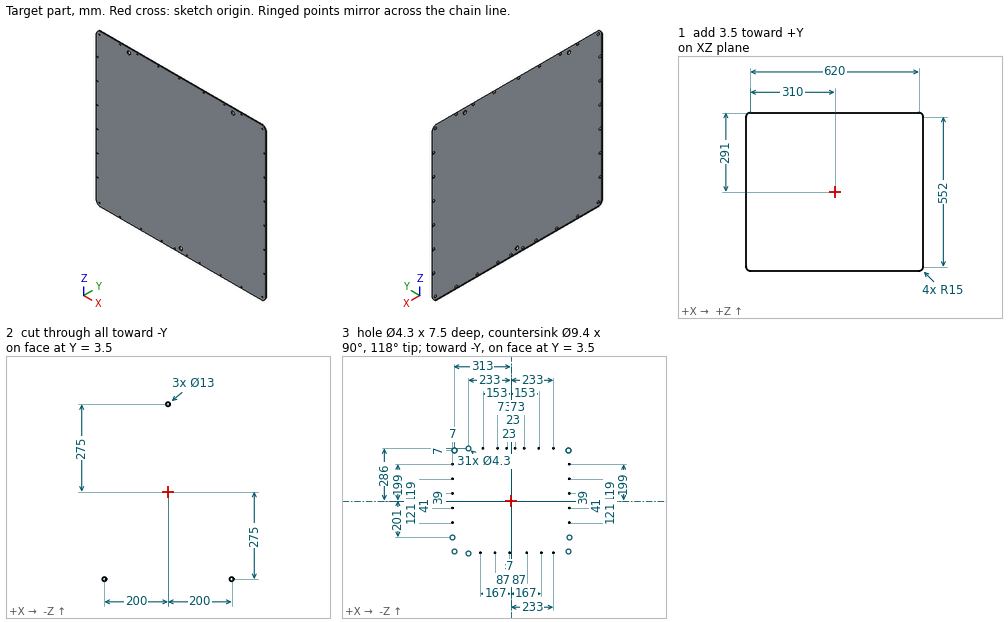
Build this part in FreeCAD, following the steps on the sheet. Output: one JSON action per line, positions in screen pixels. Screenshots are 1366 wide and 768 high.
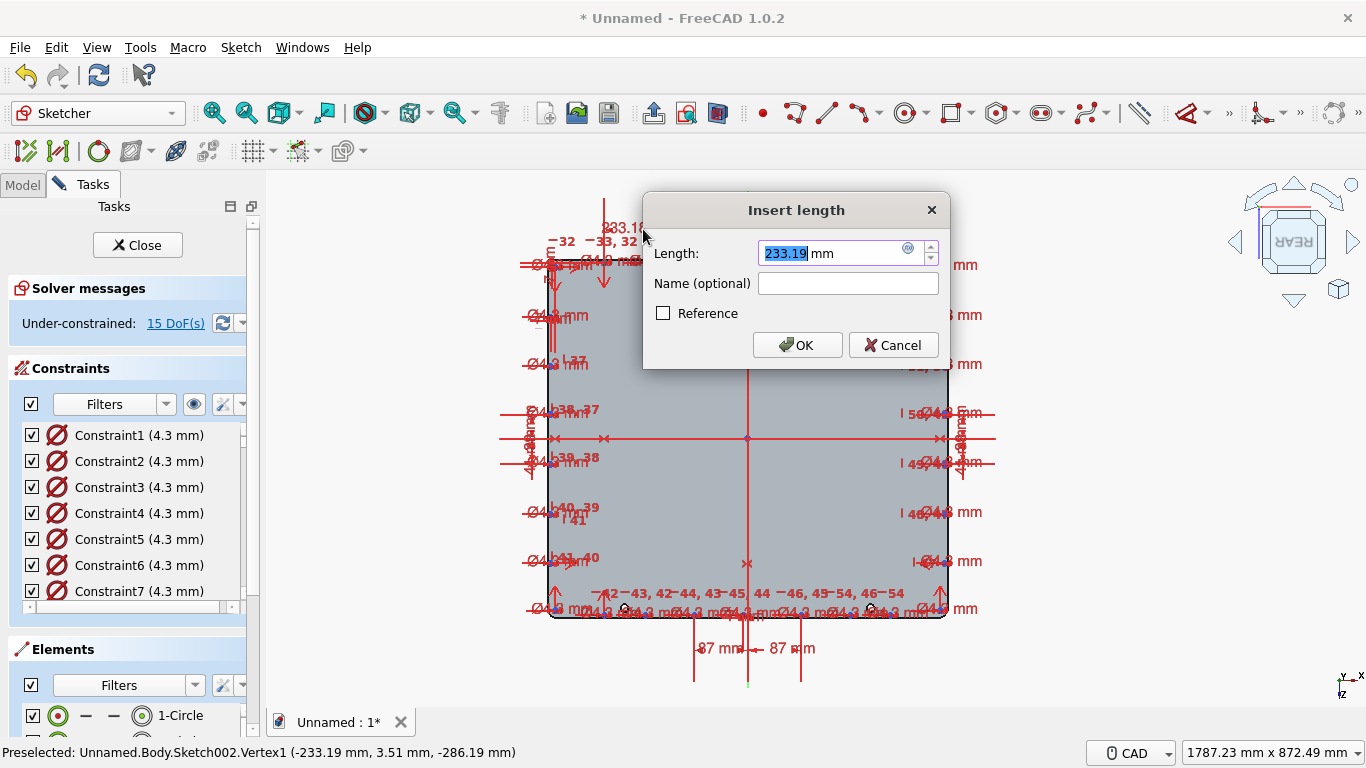
{"action": "type", "text": "233"}
{"action": "key", "text": "Return"}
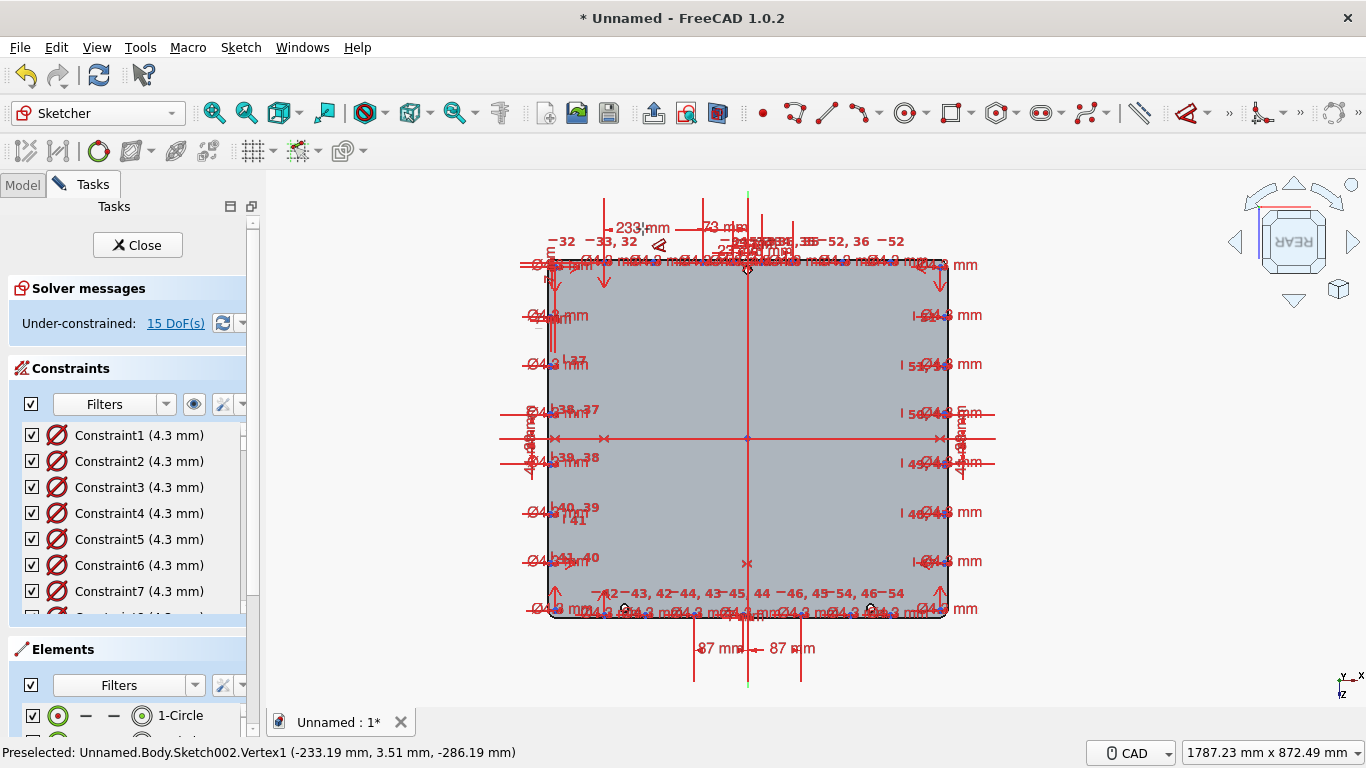
{"action": "left_click", "coordinate": [604, 263]}
{"action": "left_click", "coordinate": [570, 351]}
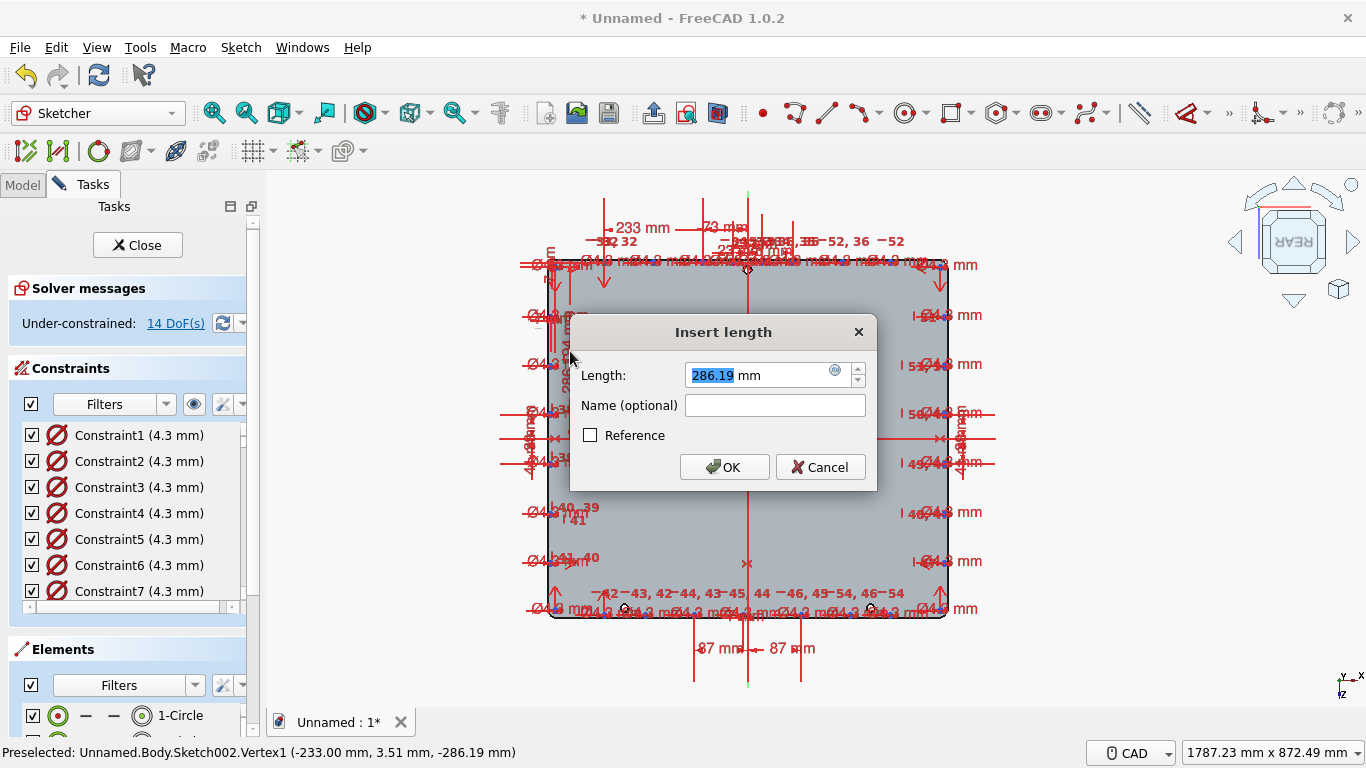
{"action": "type", "text": "286"}
{"action": "key", "text": "Return"}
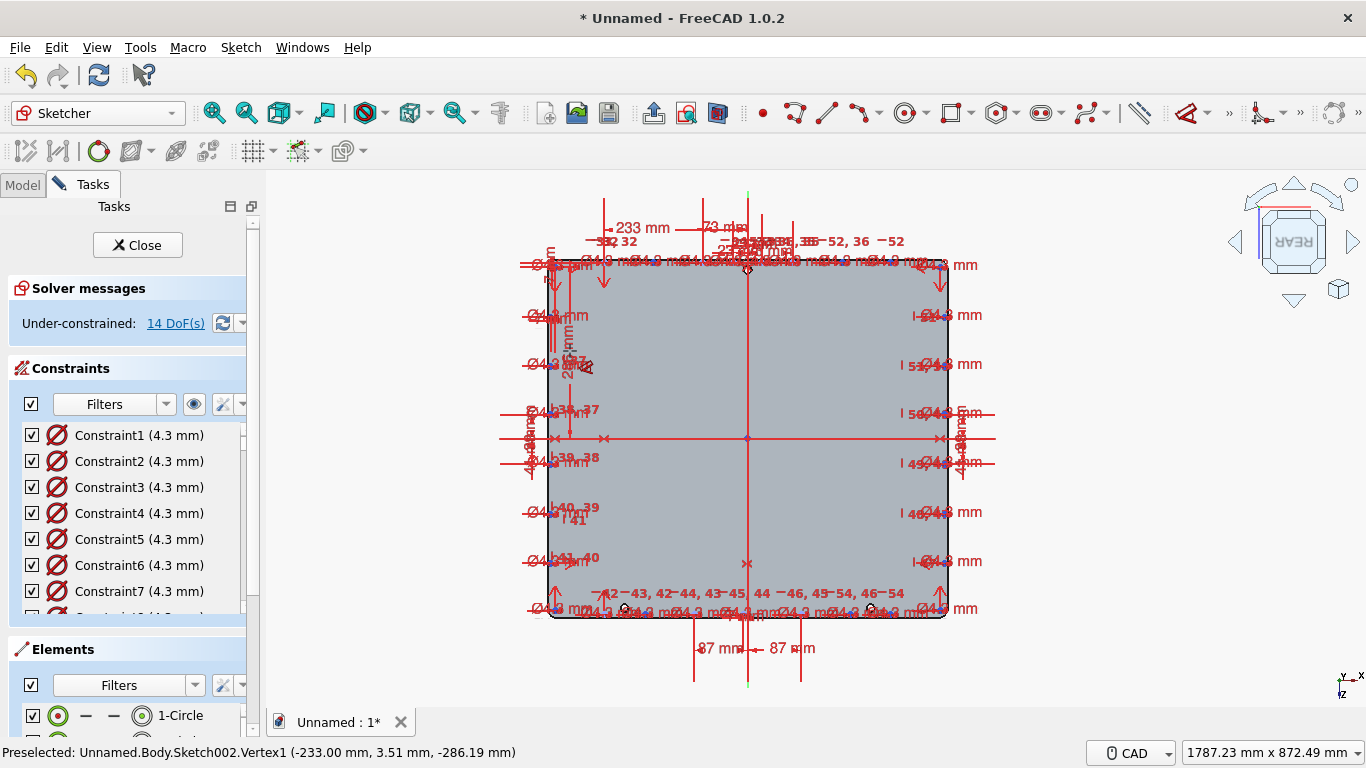
{"action": "left_click", "coordinate": [555, 267]}
{"action": "left_click", "coordinate": [651, 473]}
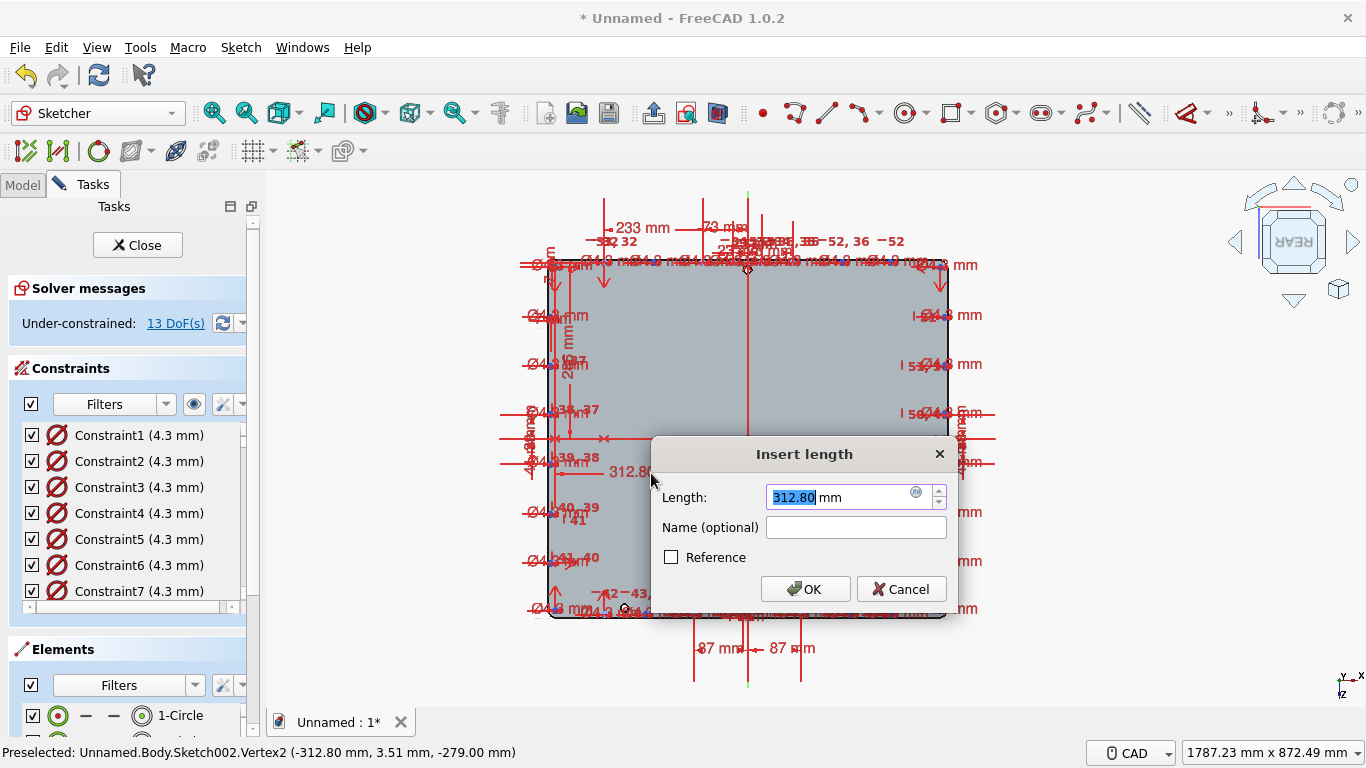
{"action": "type", "text": "313"}
{"action": "key", "text": "Return"}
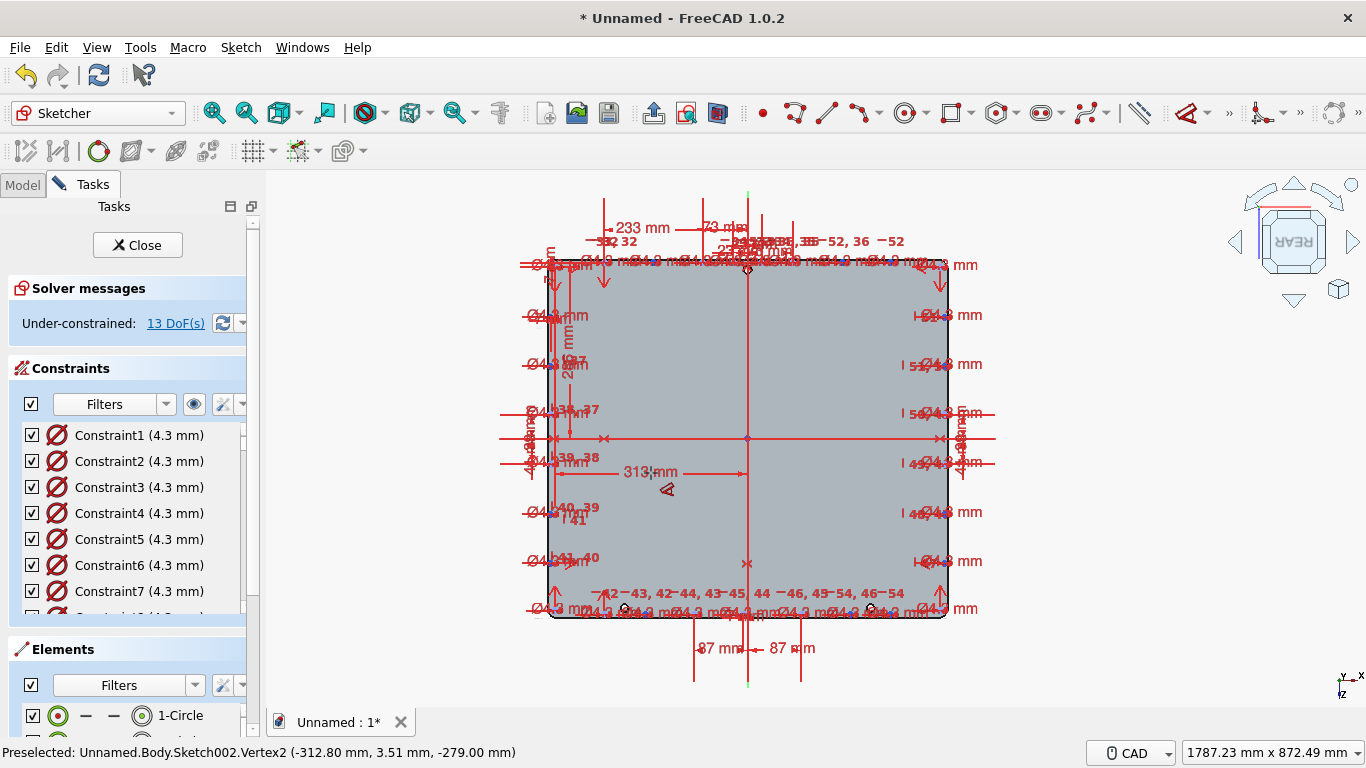
{"action": "left_click", "coordinate": [653, 263]}
{"action": "left_click", "coordinate": [722, 473]}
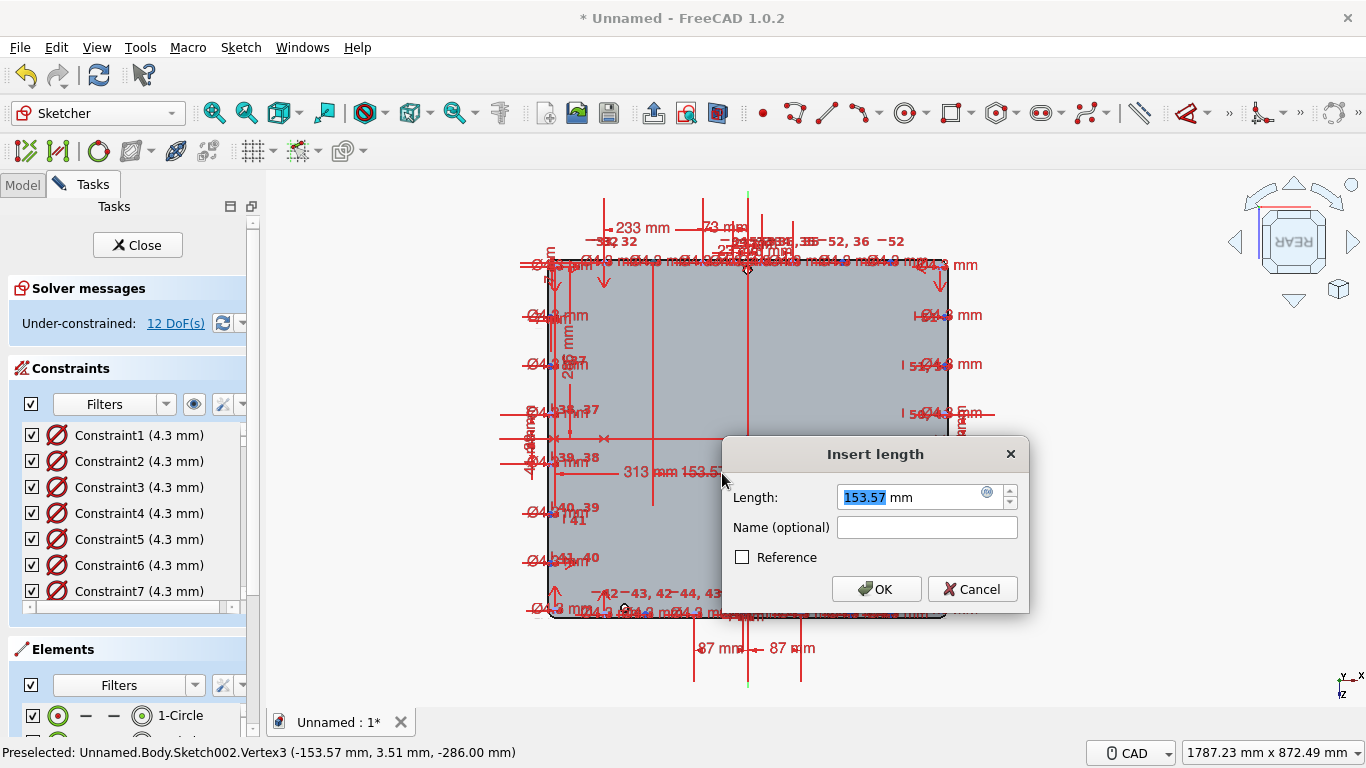
{"action": "type", "text": "153"}
{"action": "key", "text": "Return"}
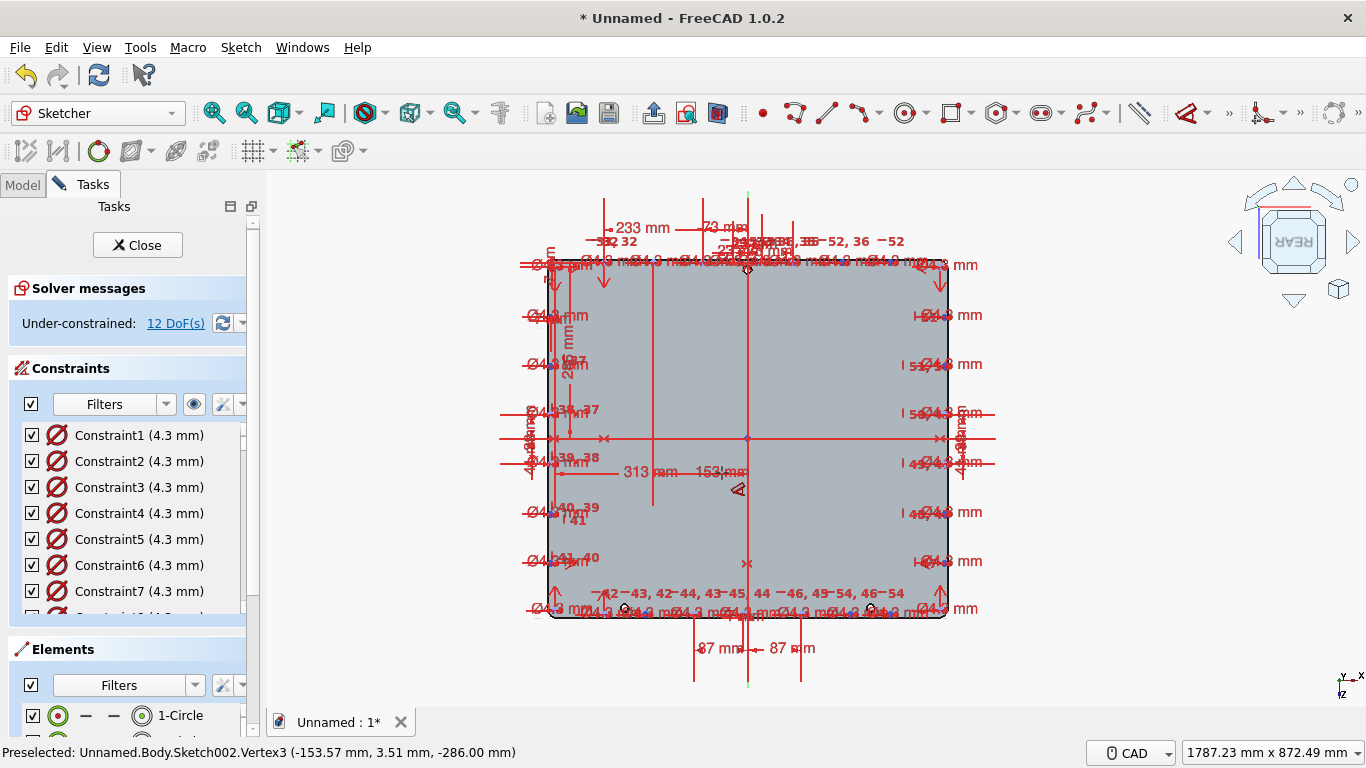
{"action": "left_click", "coordinate": [842, 263]}
{"action": "left_click", "coordinate": [828, 229]}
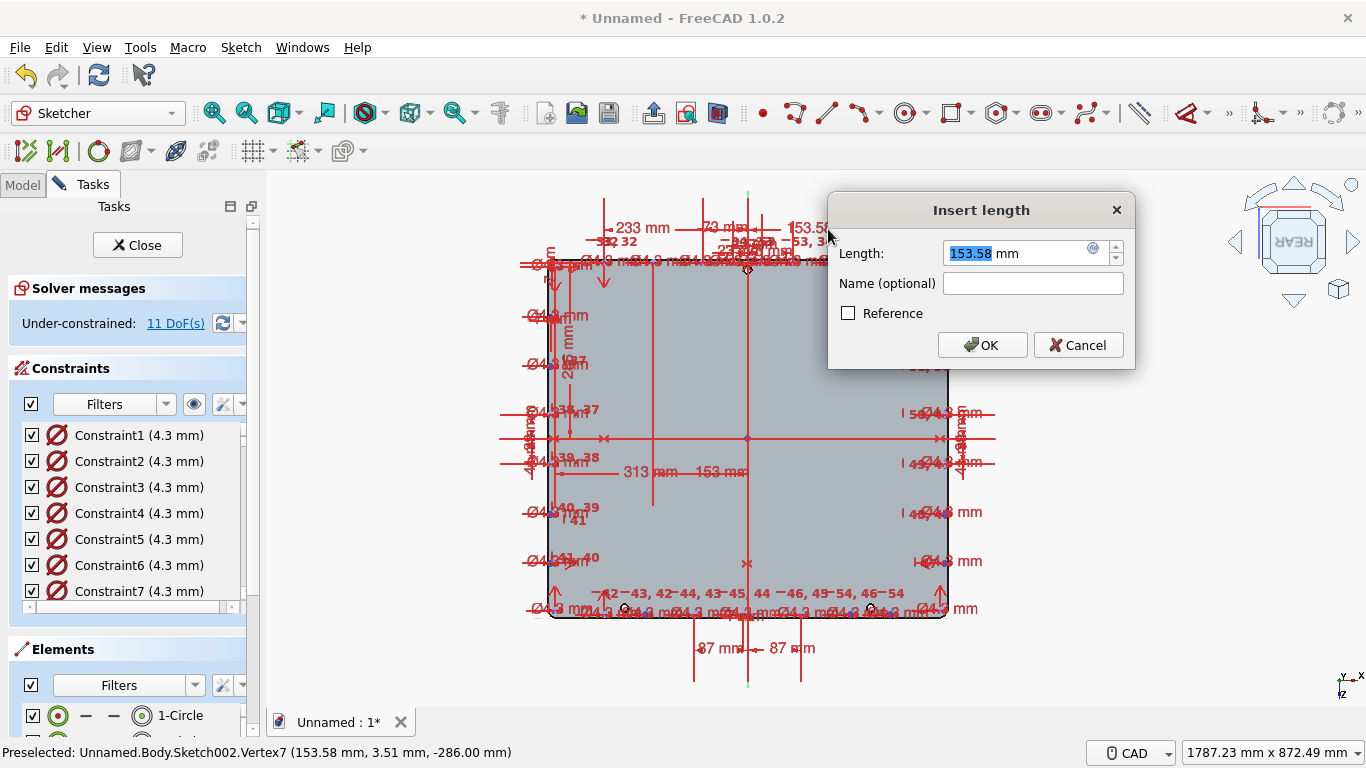
{"action": "type", "text": "153"}
{"action": "key", "text": "Return"}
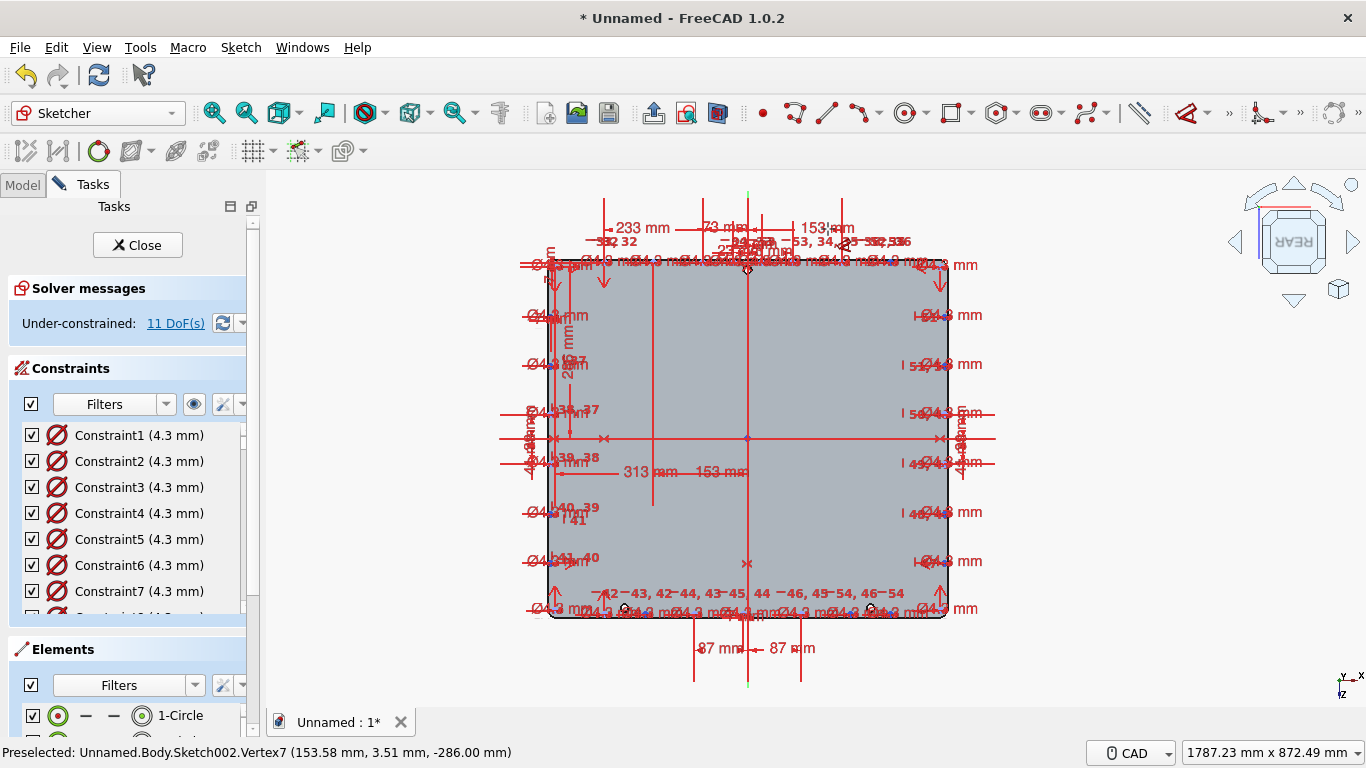
{"action": "left_click", "coordinate": [551, 317]}
{"action": "left_click", "coordinate": [517, 378]}